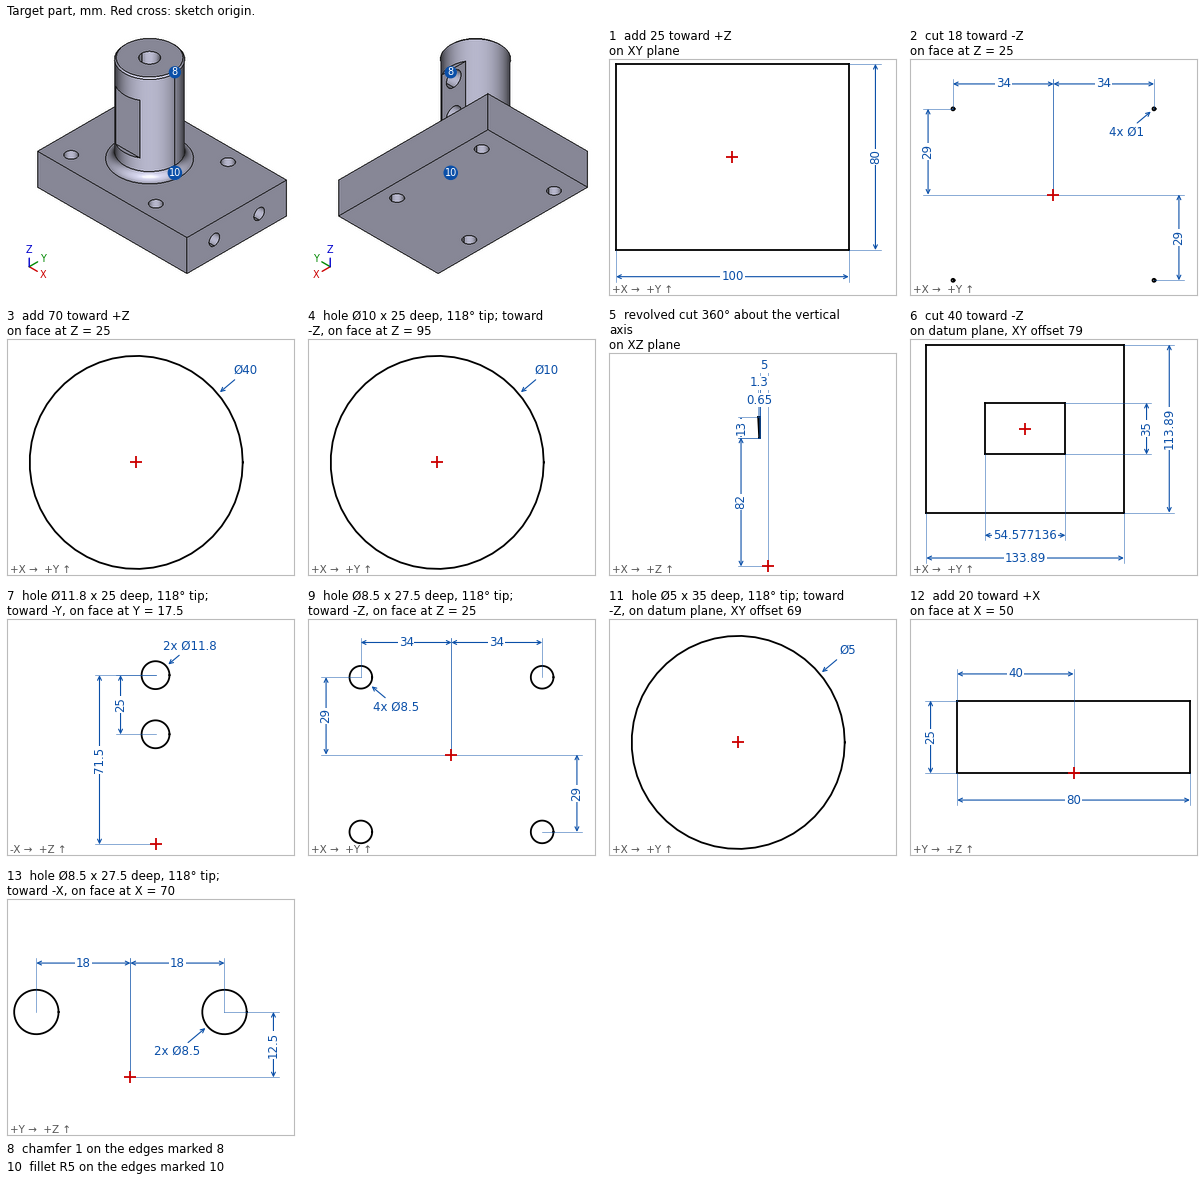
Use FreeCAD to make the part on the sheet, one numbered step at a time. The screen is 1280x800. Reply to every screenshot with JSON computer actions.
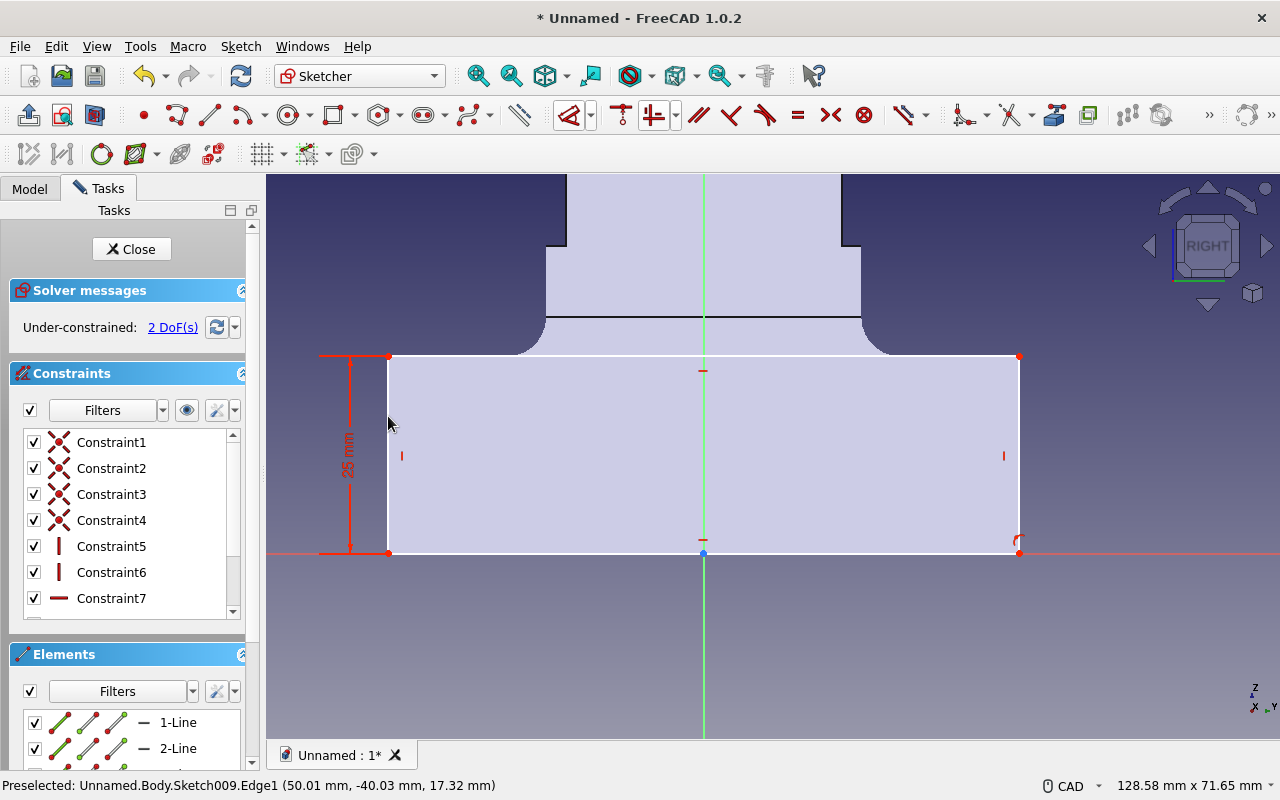
{"action": "left_click", "coordinate": [577, 554]}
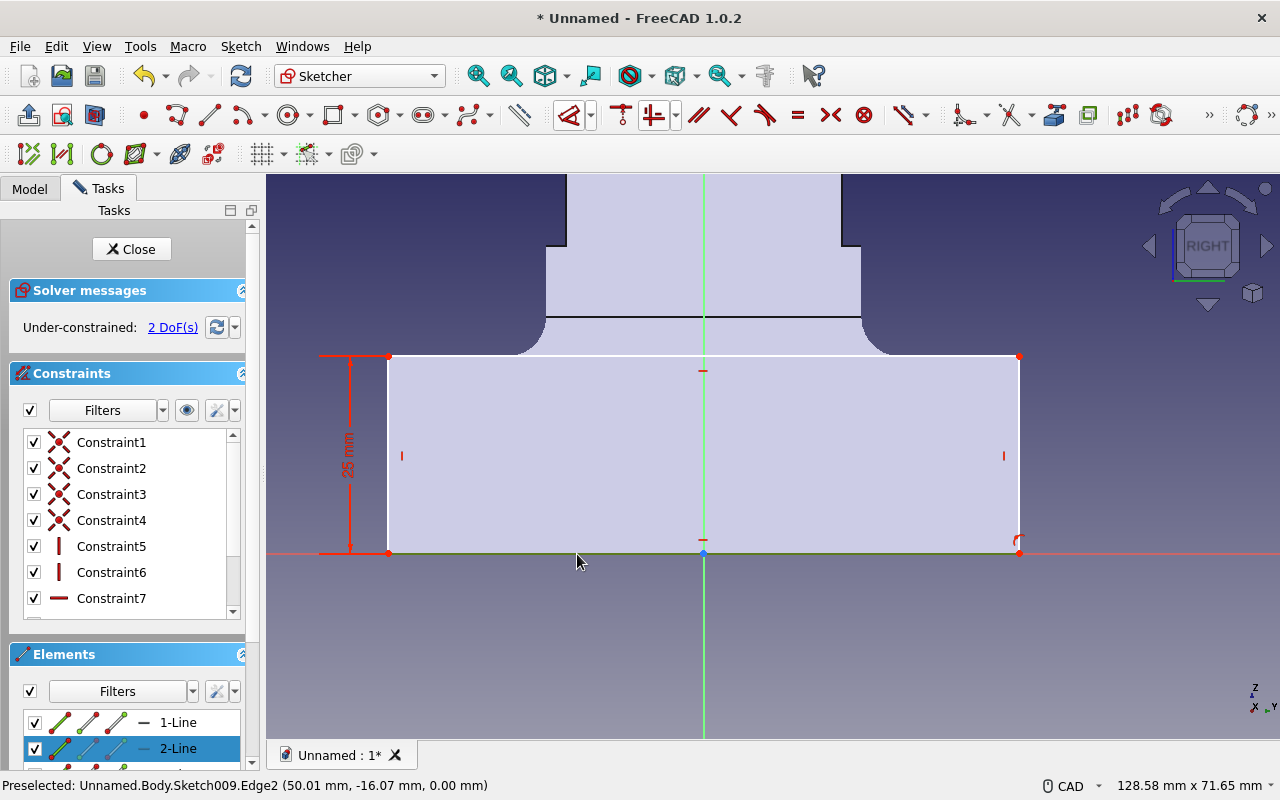
{"action": "key", "text": "l"}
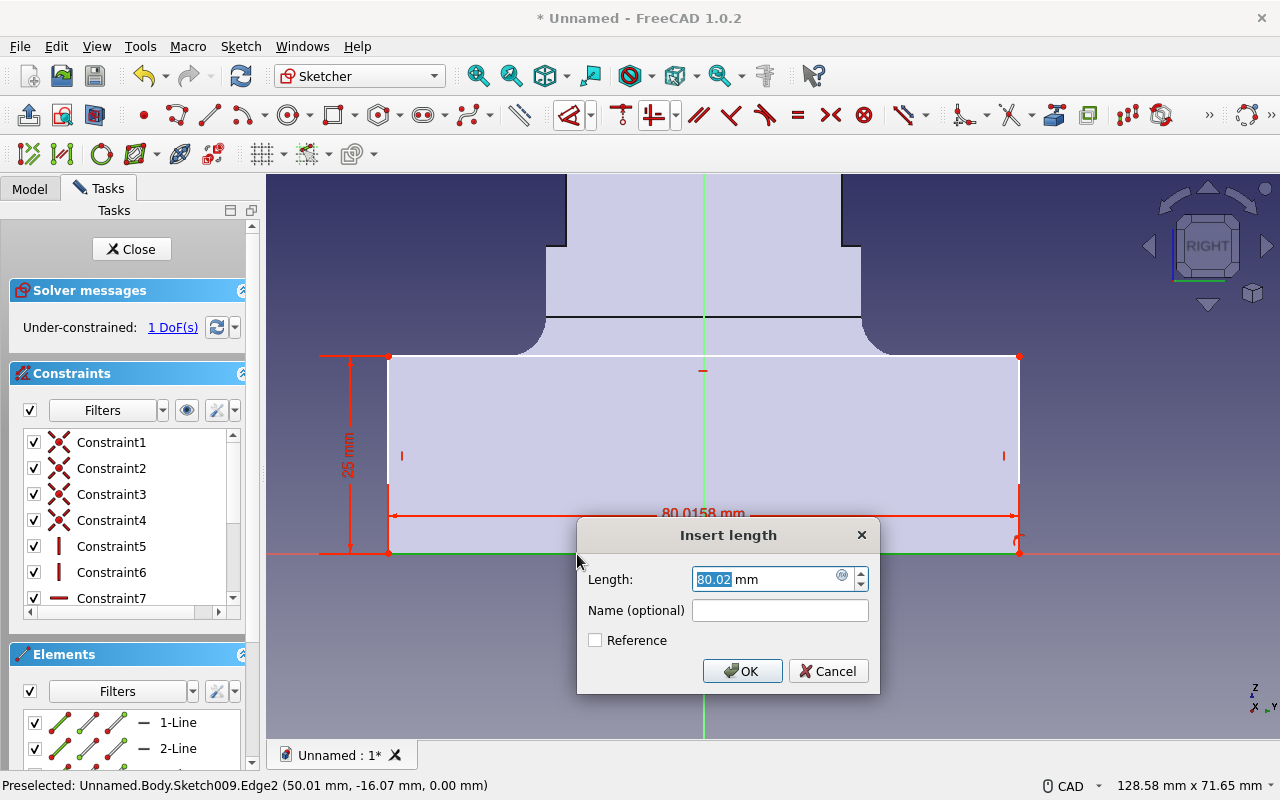
{"action": "type", "text": "80"}
{"action": "key", "text": "Return"}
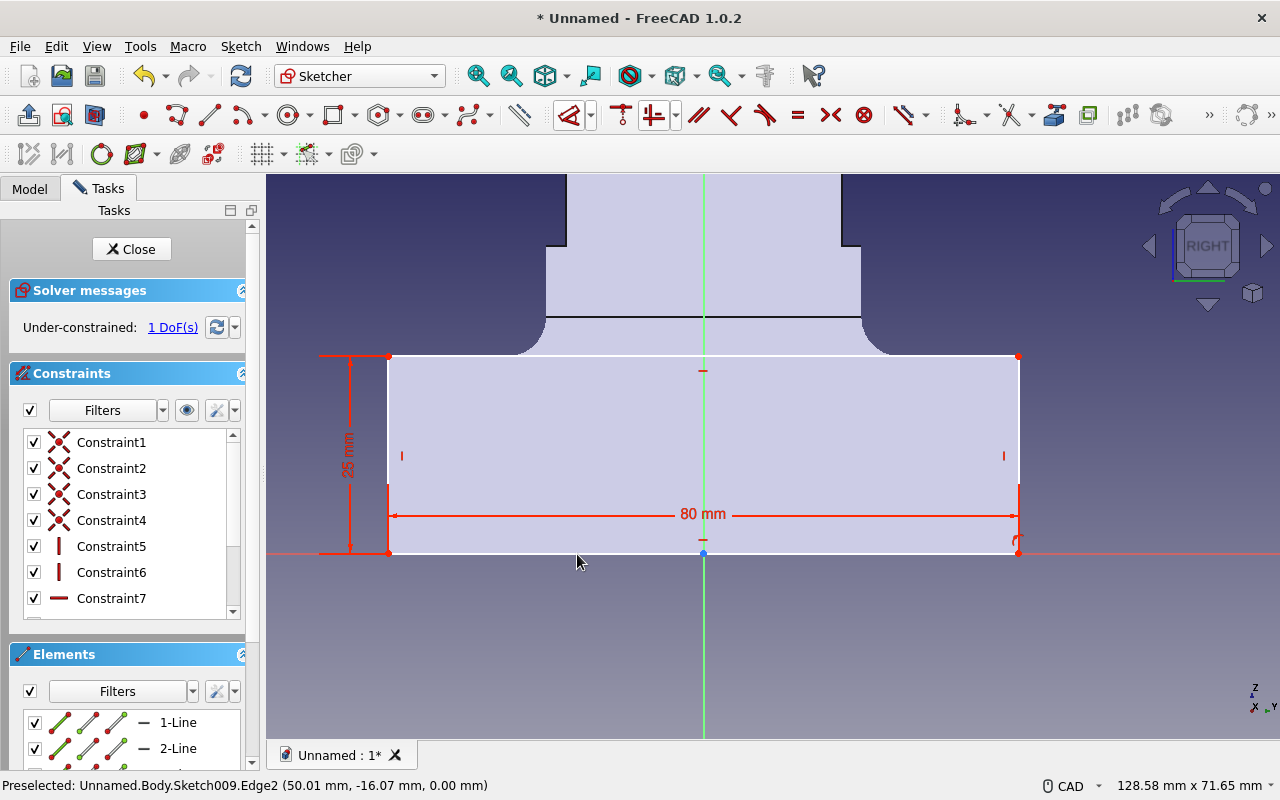
{"action": "left_click", "coordinate": [388, 356]}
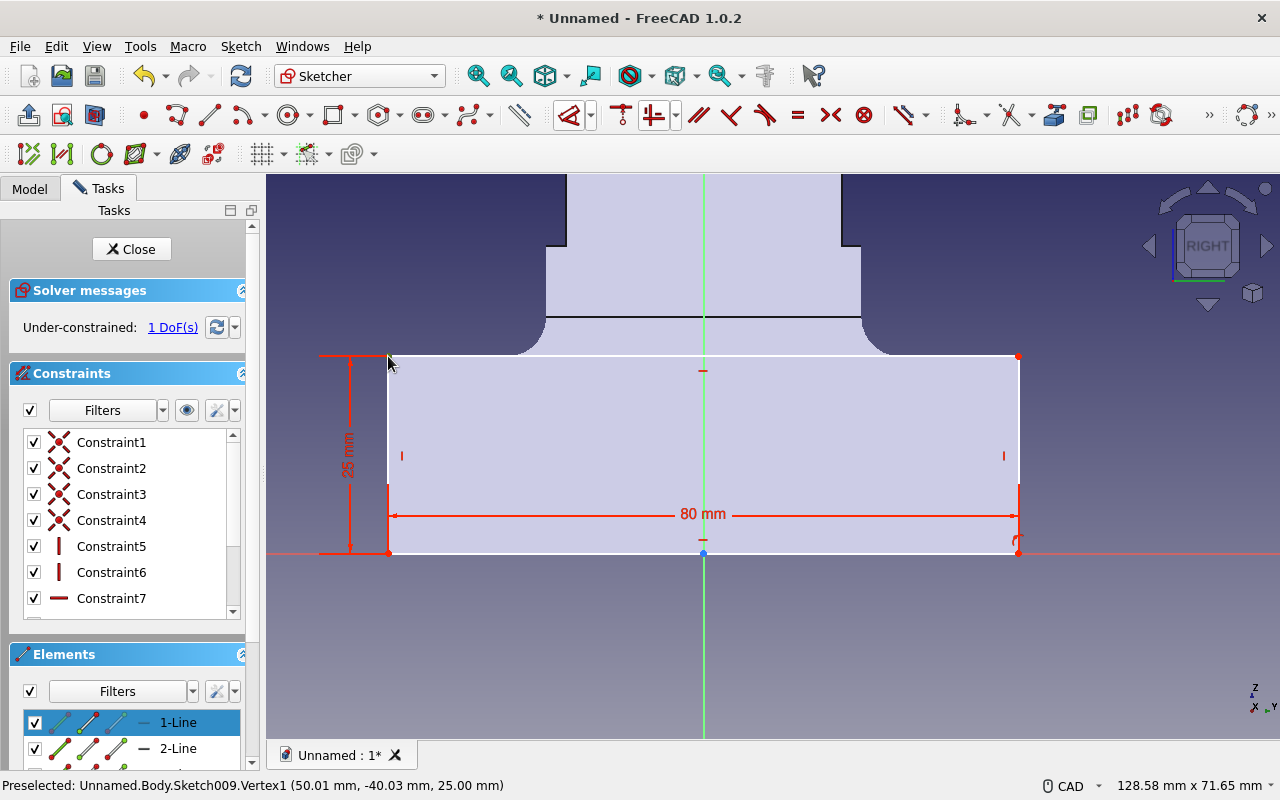
{"action": "left_click", "coordinate": [590, 116]}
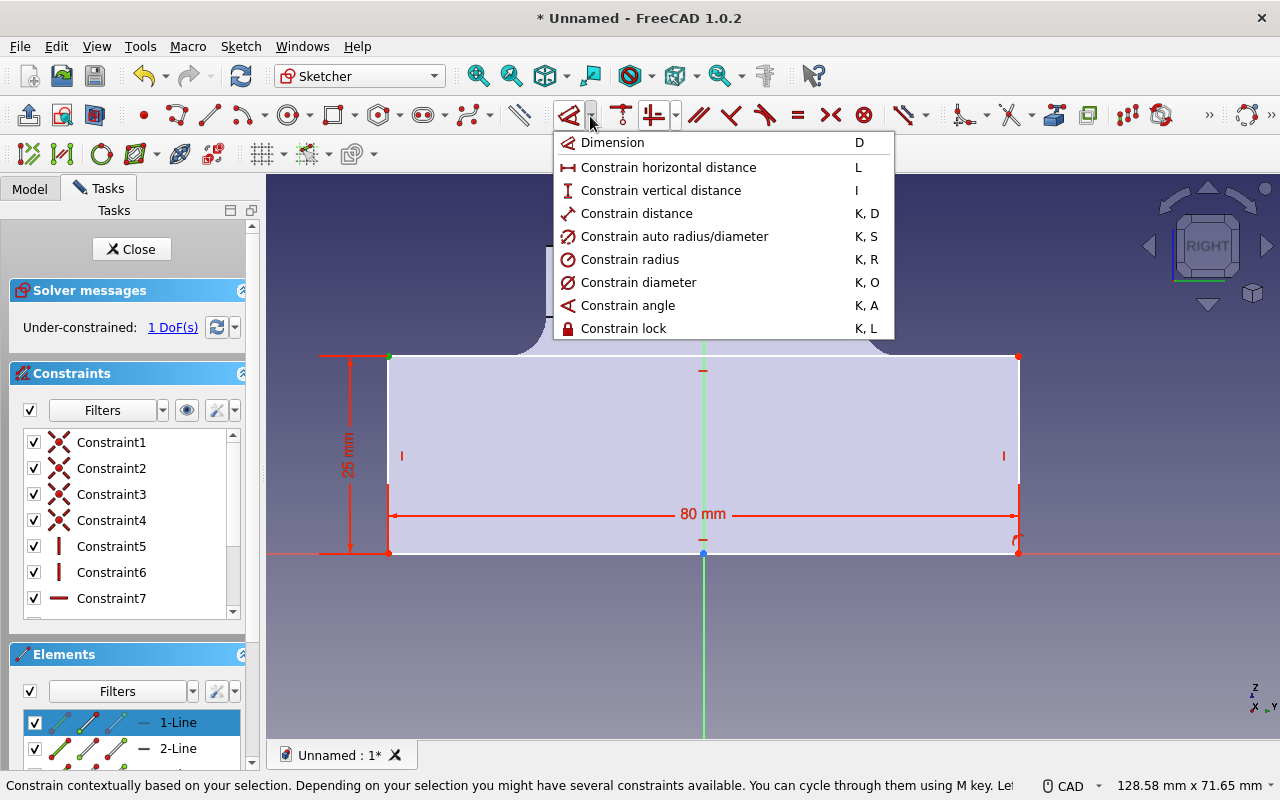
{"action": "left_click", "coordinate": [724, 168]}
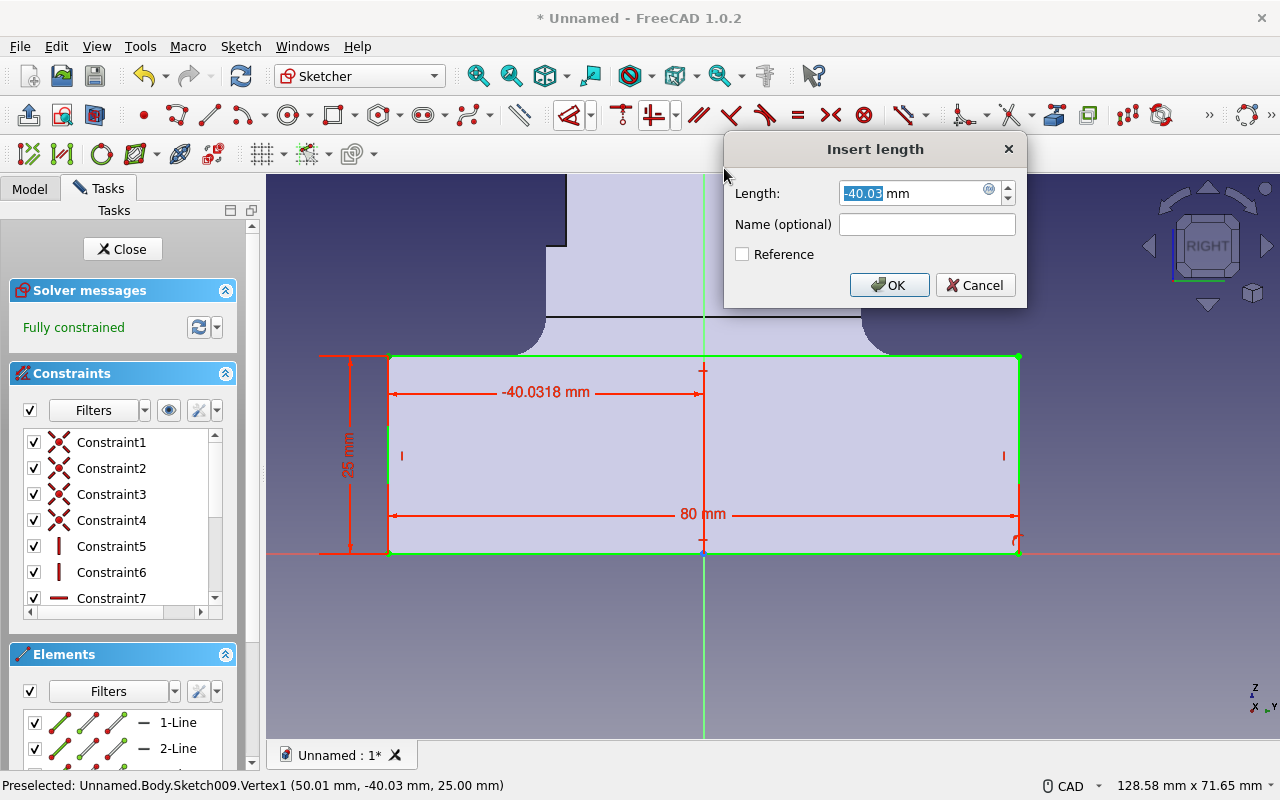
{"action": "type", "text": "-40"}
{"action": "key", "text": "Return"}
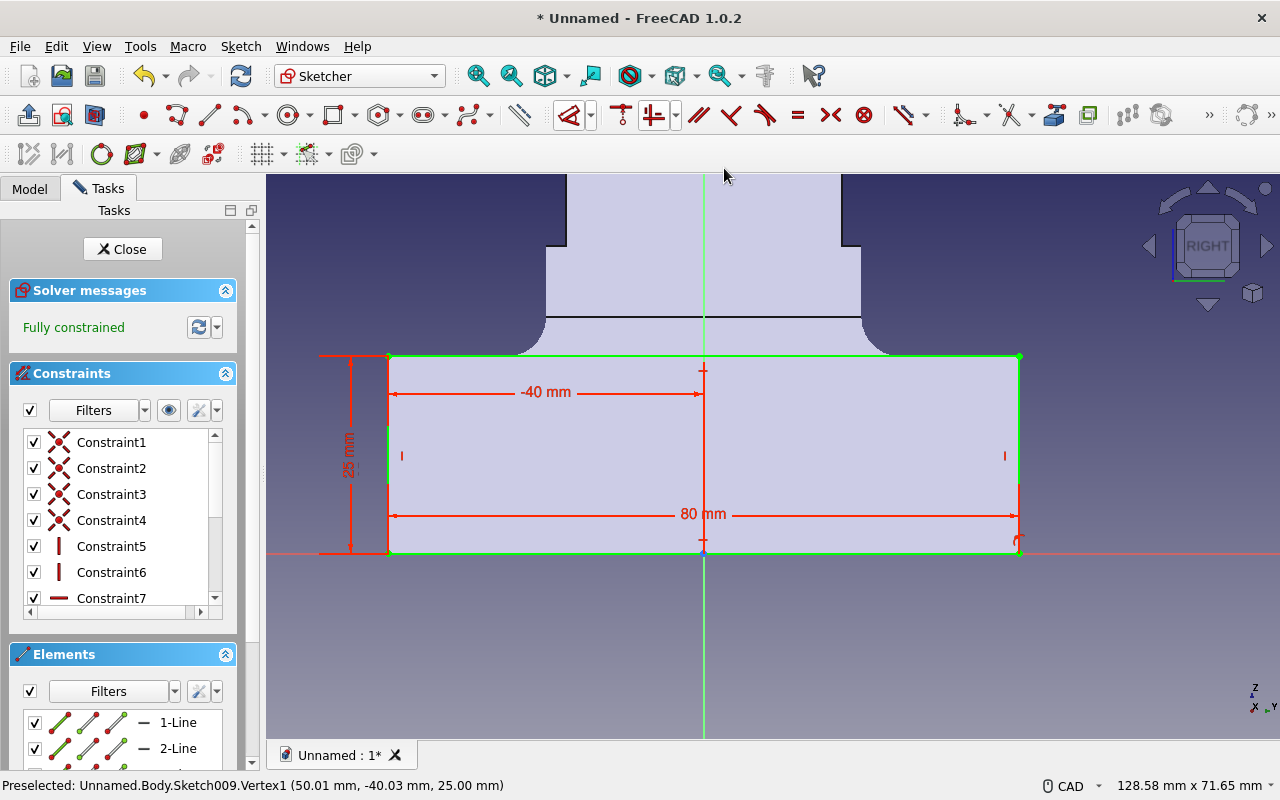
{"action": "left_click", "coordinate": [123, 249]}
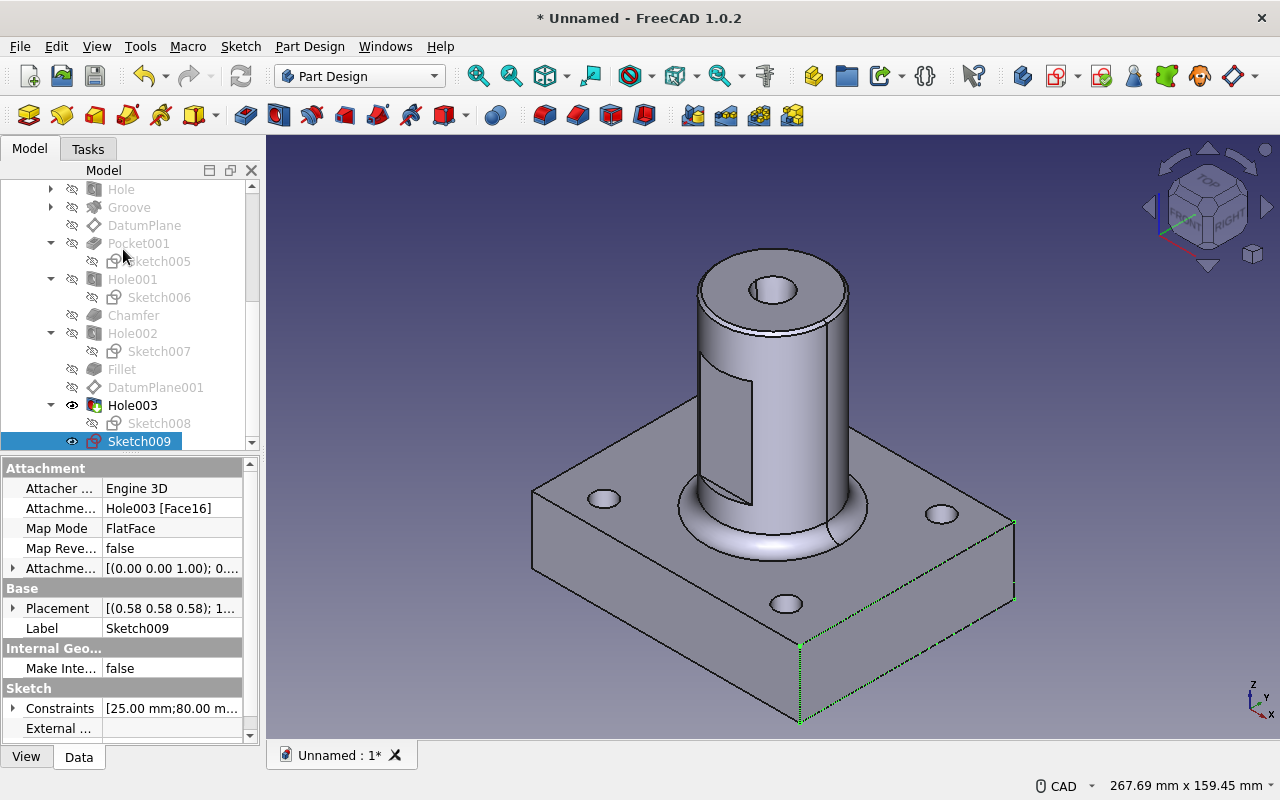
{"action": "left_click", "coordinate": [29, 116]}